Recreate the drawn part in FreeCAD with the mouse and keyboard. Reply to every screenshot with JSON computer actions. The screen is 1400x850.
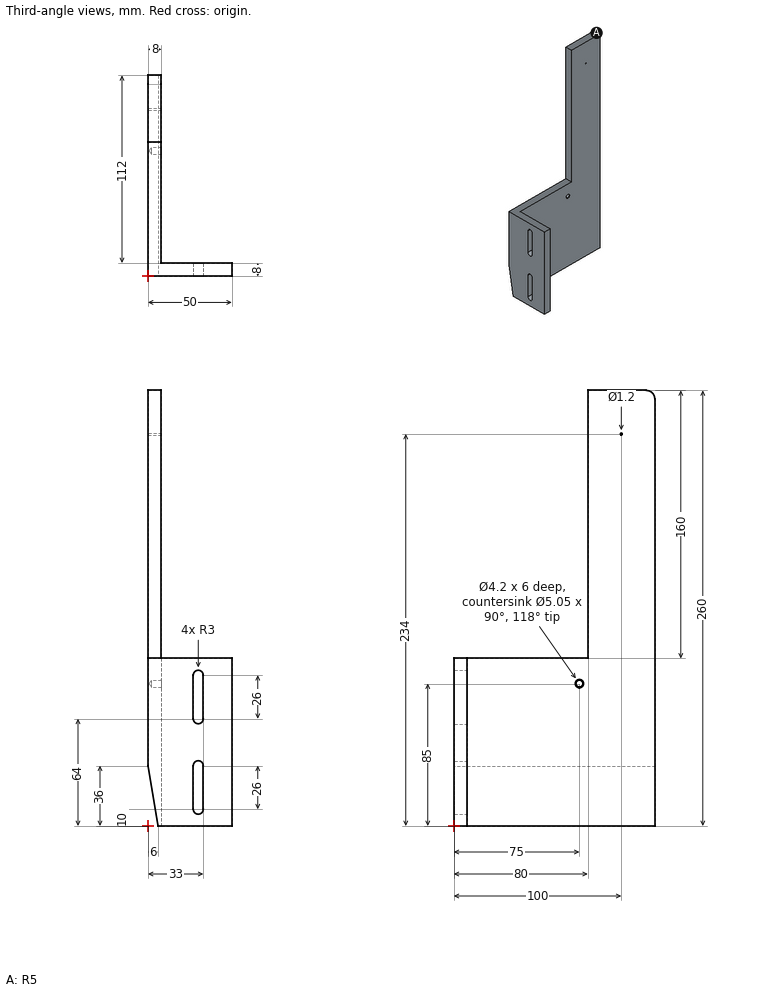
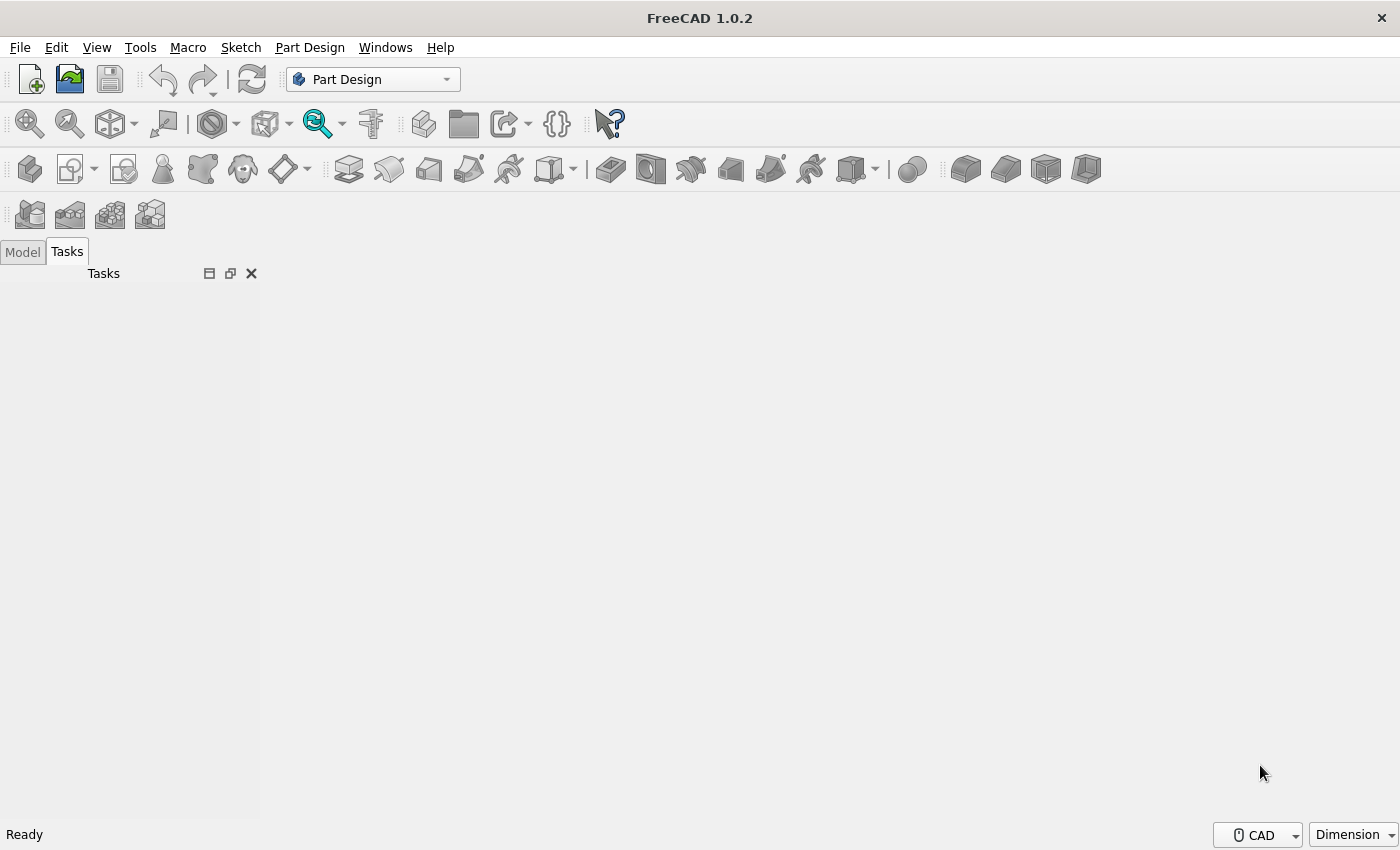
{"action": "left_click", "coordinate": [30, 80]}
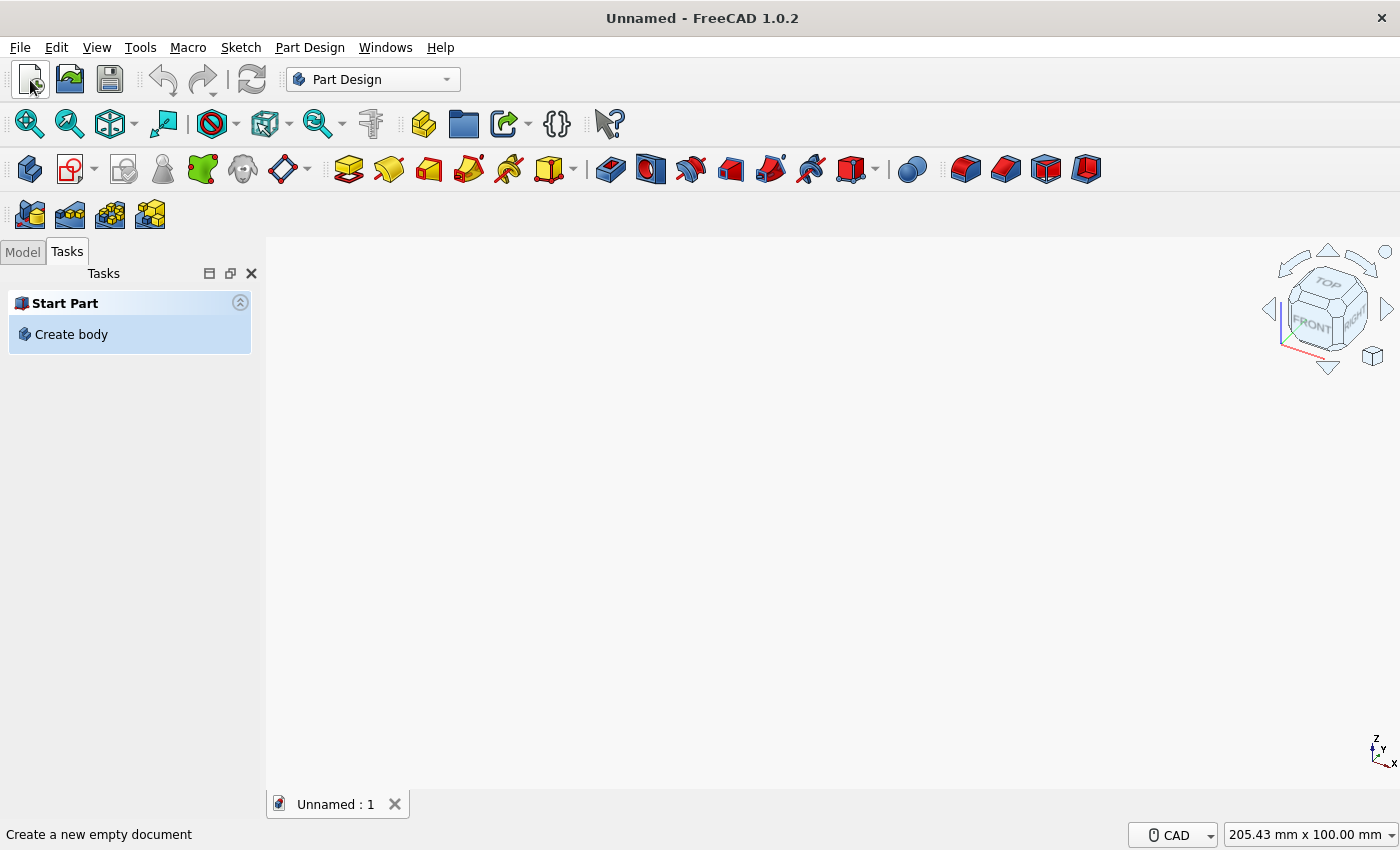
{"action": "left_click", "coordinate": [70, 170]}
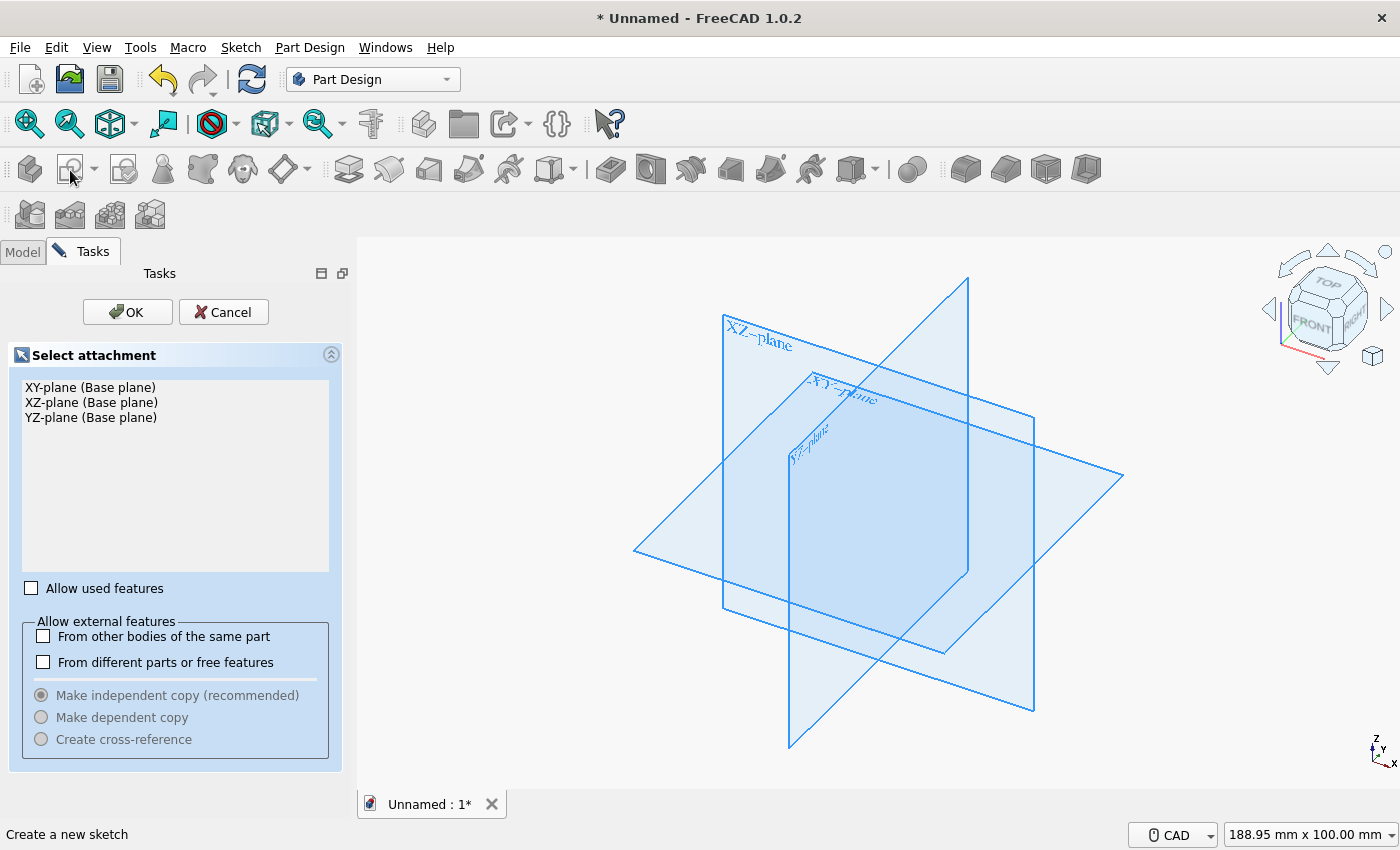
{"action": "left_click", "coordinate": [82, 388]}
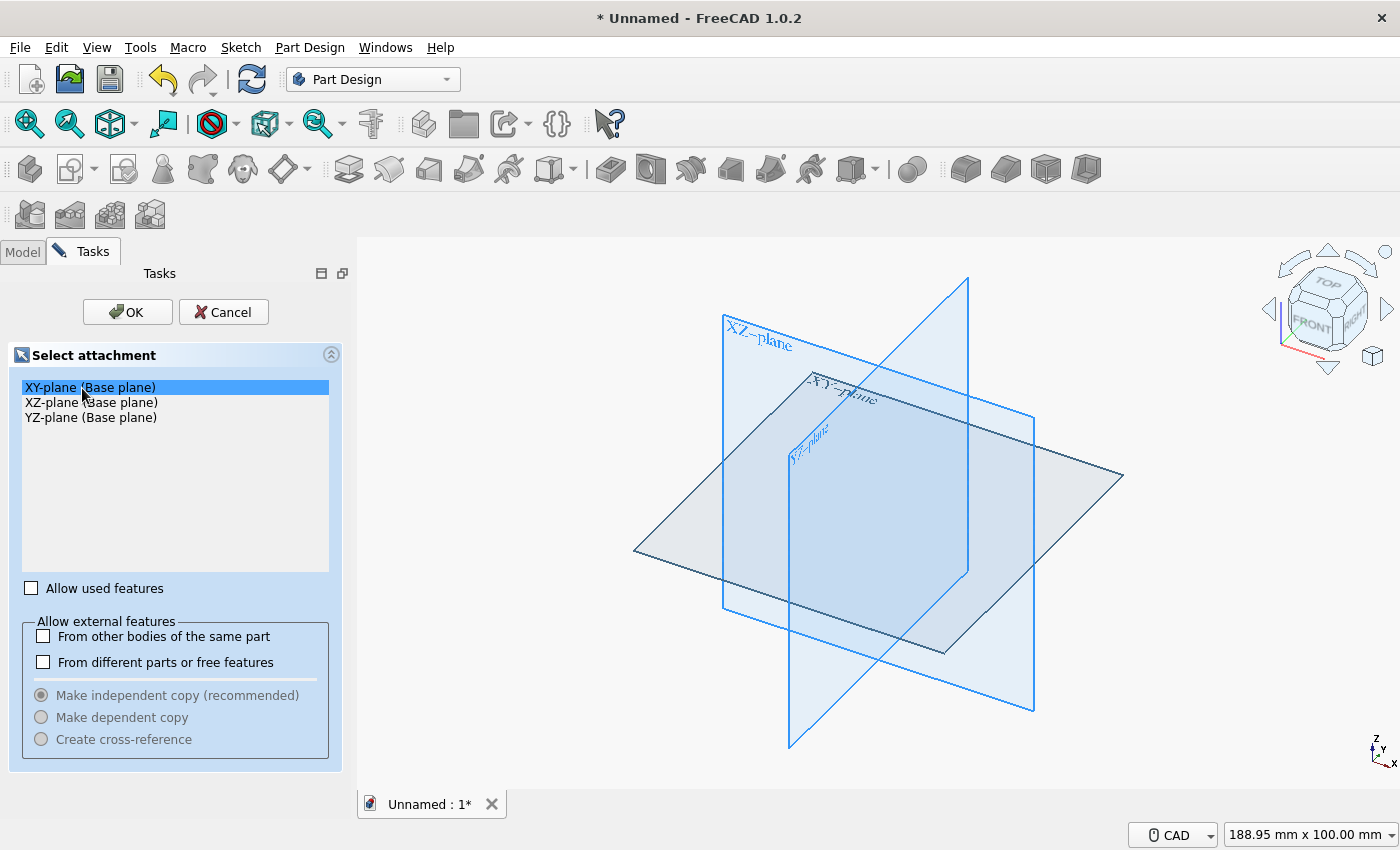
{"action": "left_click", "coordinate": [128, 312]}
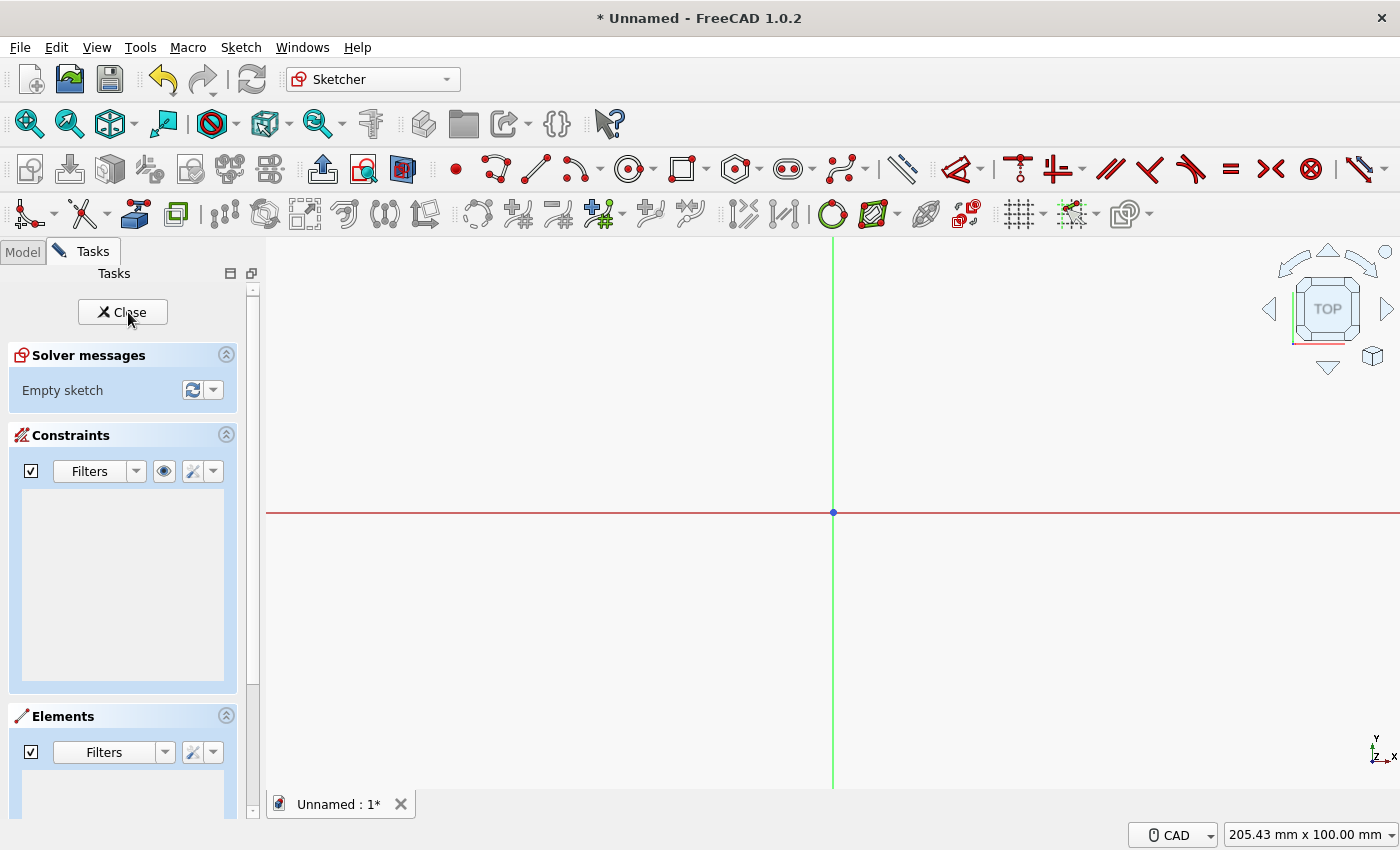
{"action": "scroll", "coordinate": [596, 761], "scroll_direction": "down", "scroll_amount": 4}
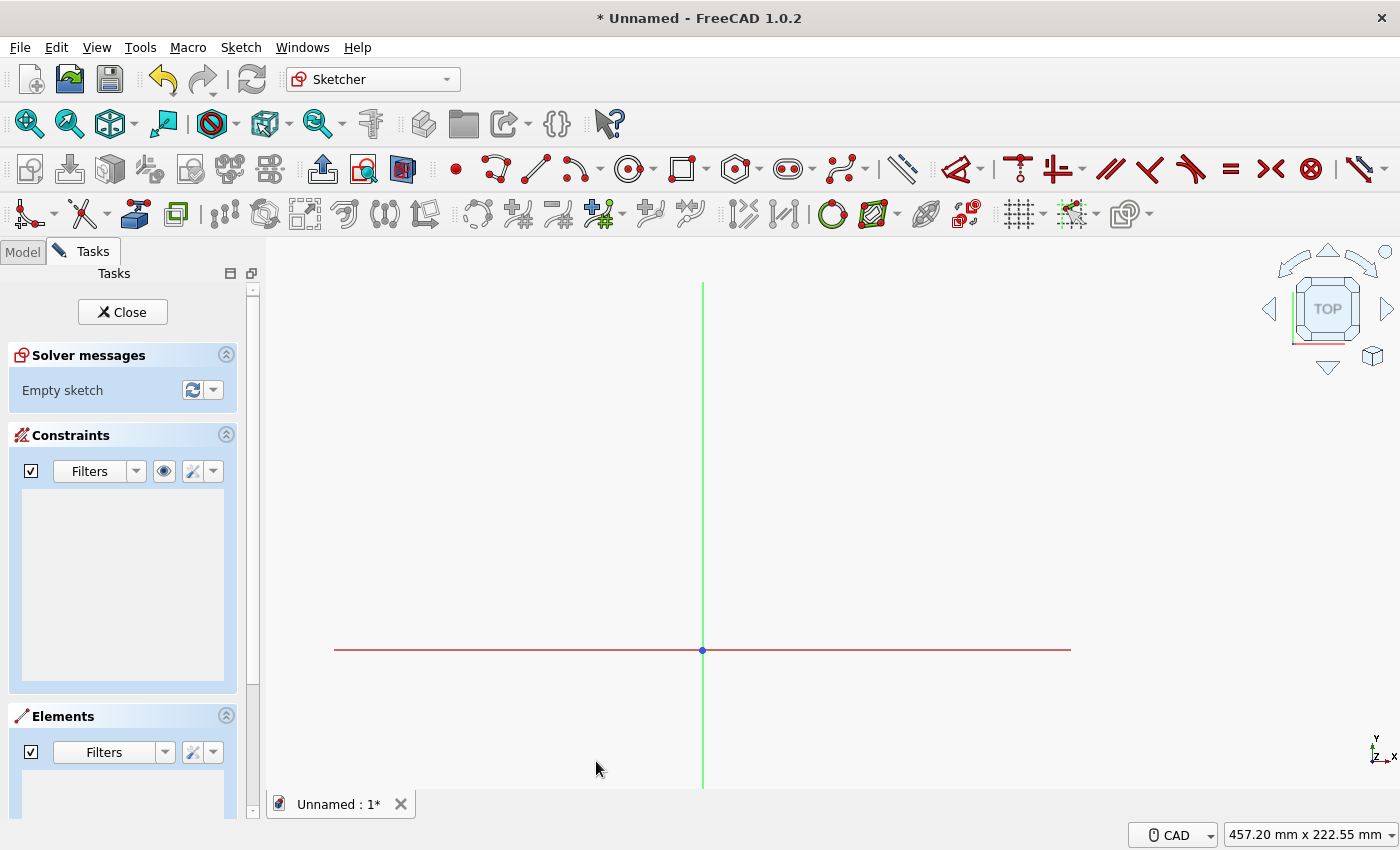
{"action": "left_click", "coordinate": [496, 170]}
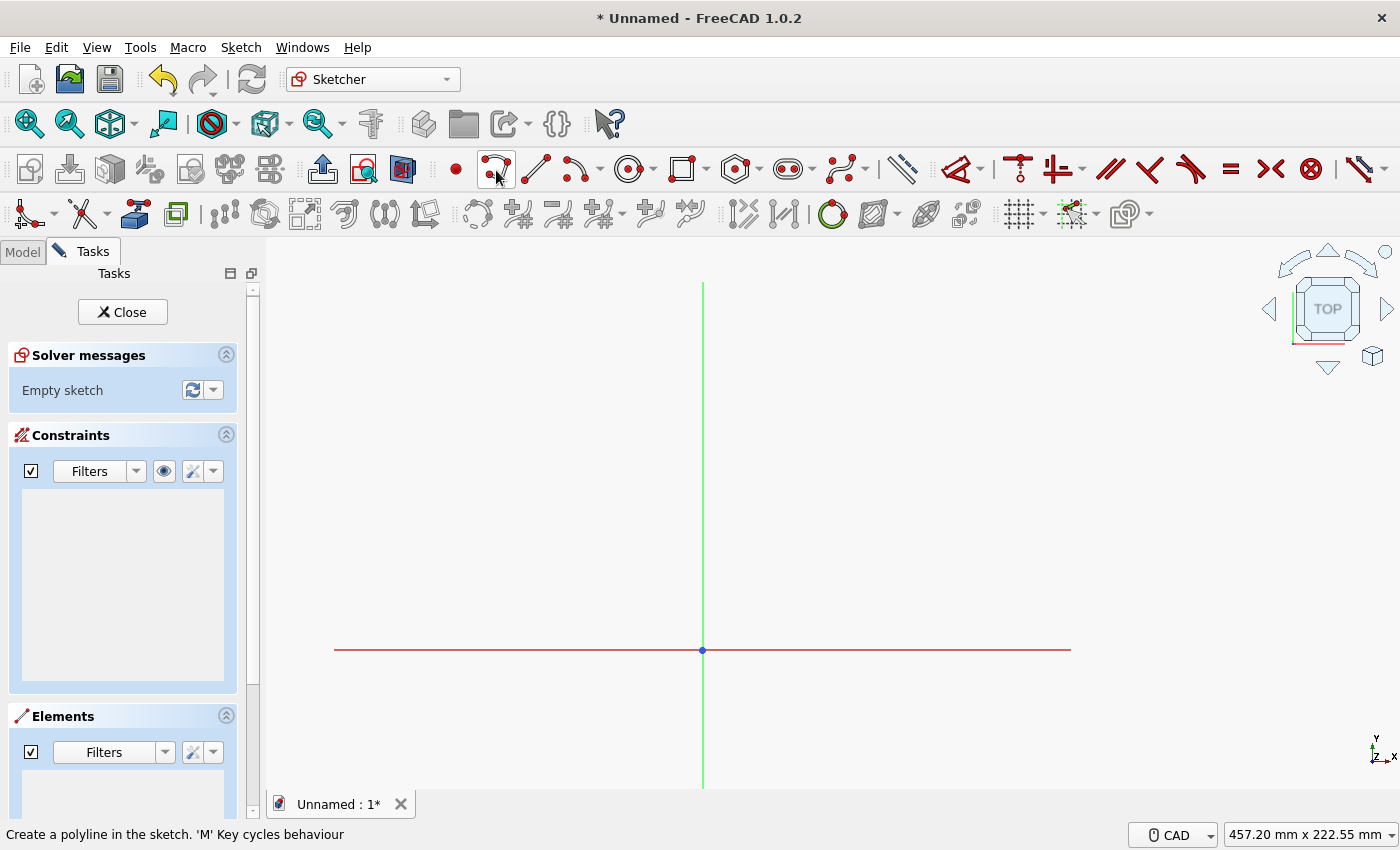
{"action": "left_click", "coordinate": [703, 650]}
{"action": "left_click", "coordinate": [827, 641]}
{"action": "left_click", "coordinate": [827, 630]}
{"action": "left_click", "coordinate": [722, 630]}
{"action": "left_click", "coordinate": [722, 352]}
{"action": "left_click", "coordinate": [712, 352]}
{"action": "left_click", "coordinate": [703, 650]}
{"action": "key", "text": "Escape"}
{"action": "key", "text": "Escape"}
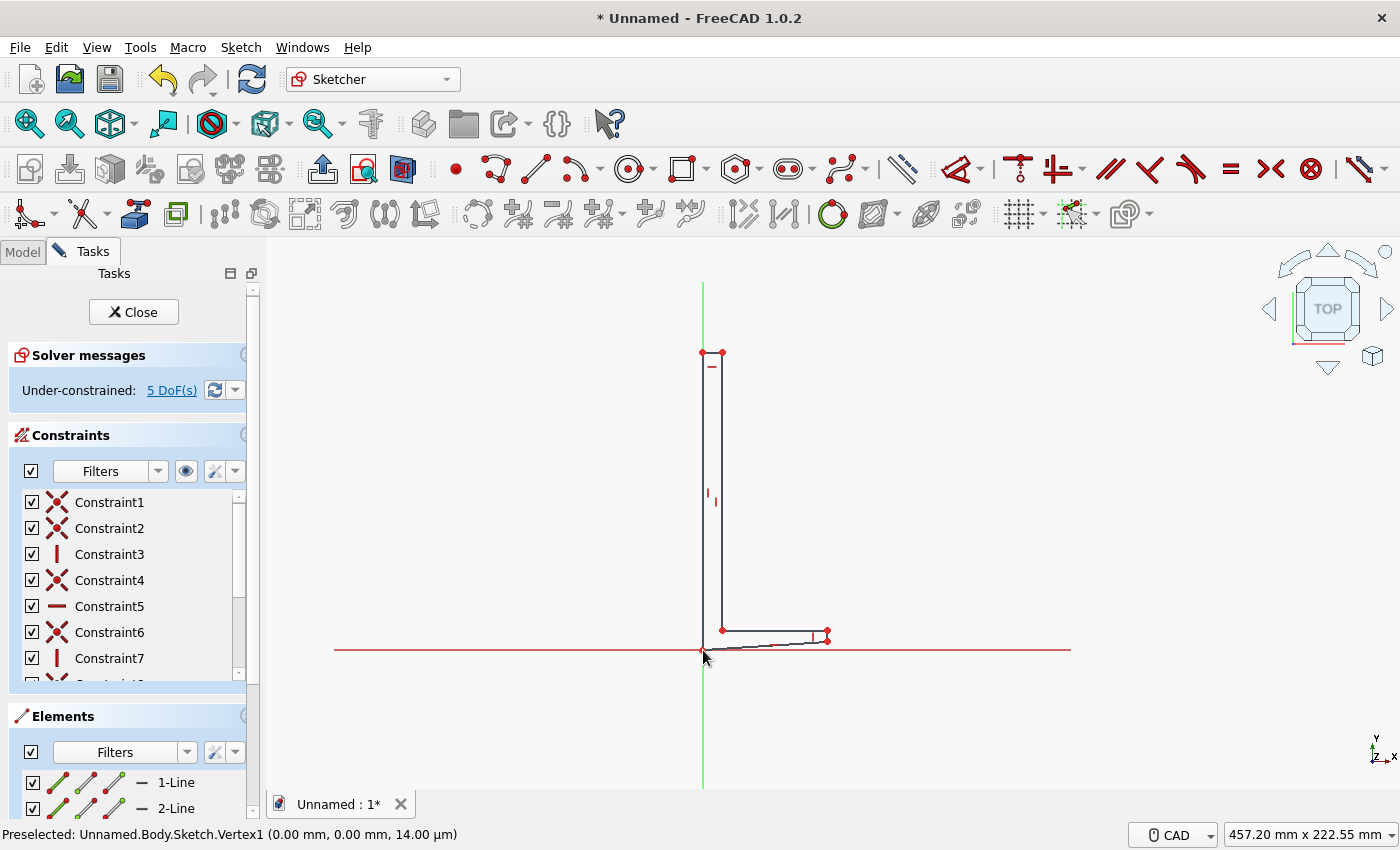
{"action": "left_click", "coordinate": [740, 648]}